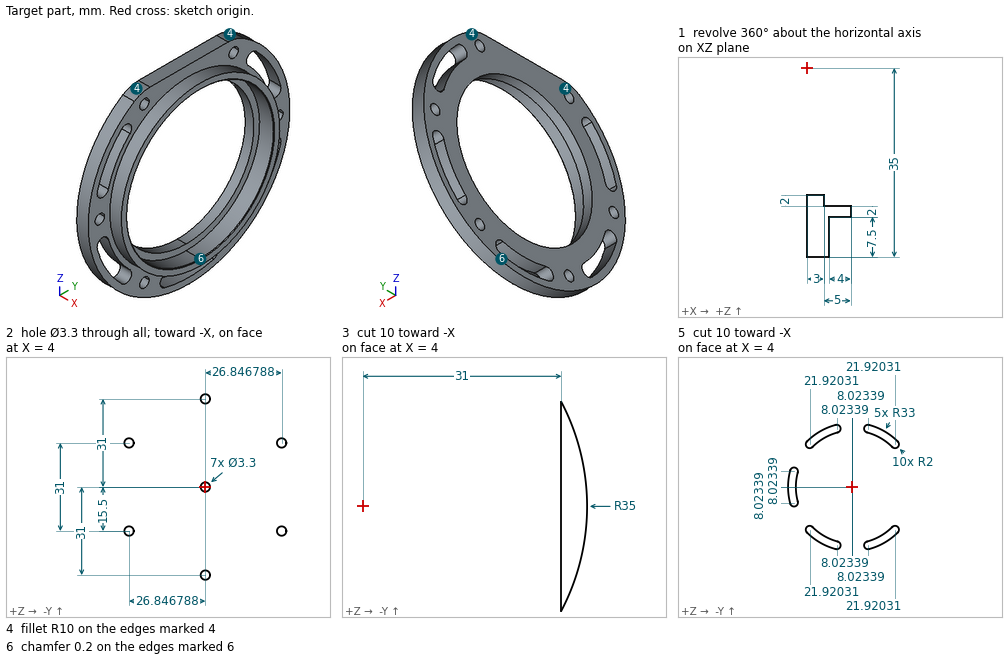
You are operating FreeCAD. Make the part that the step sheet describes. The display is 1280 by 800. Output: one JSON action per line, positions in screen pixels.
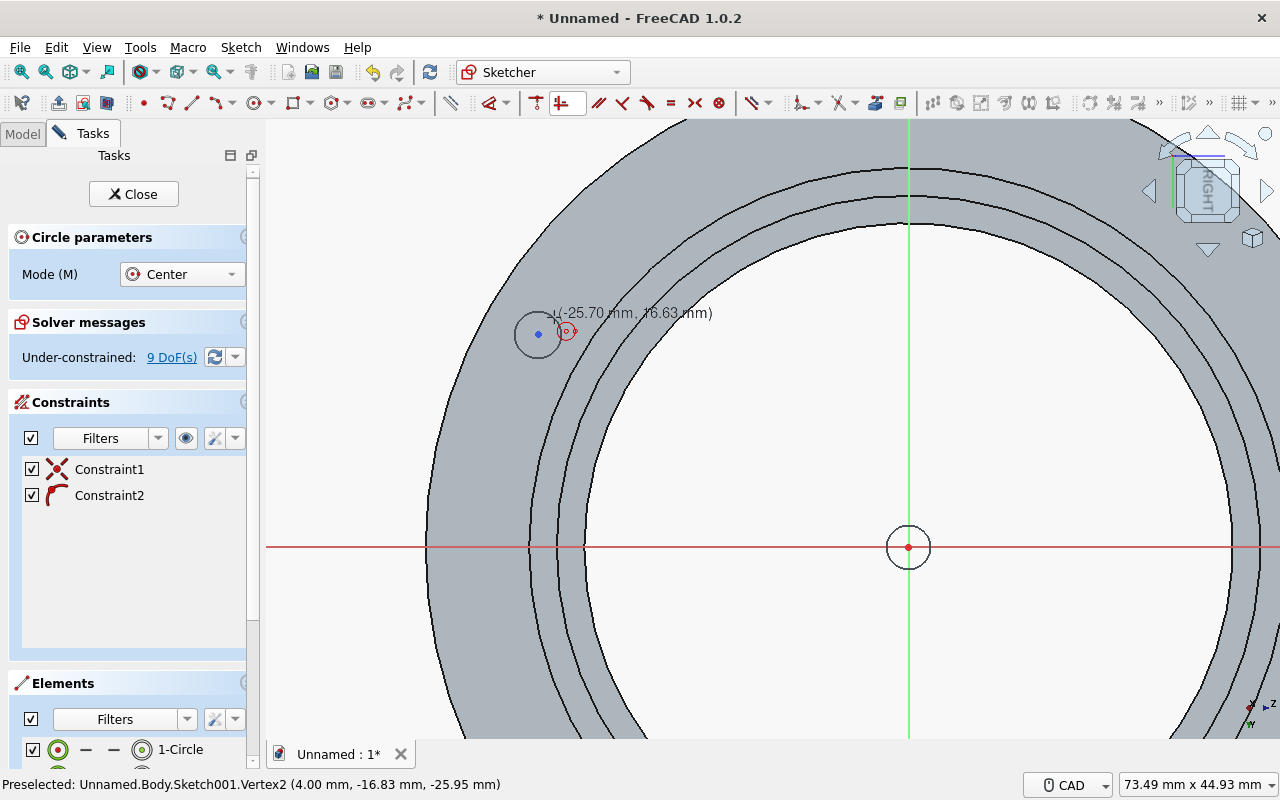
{"action": "scroll", "coordinate": [538, 332], "scroll_direction": "down", "scroll_amount": 4}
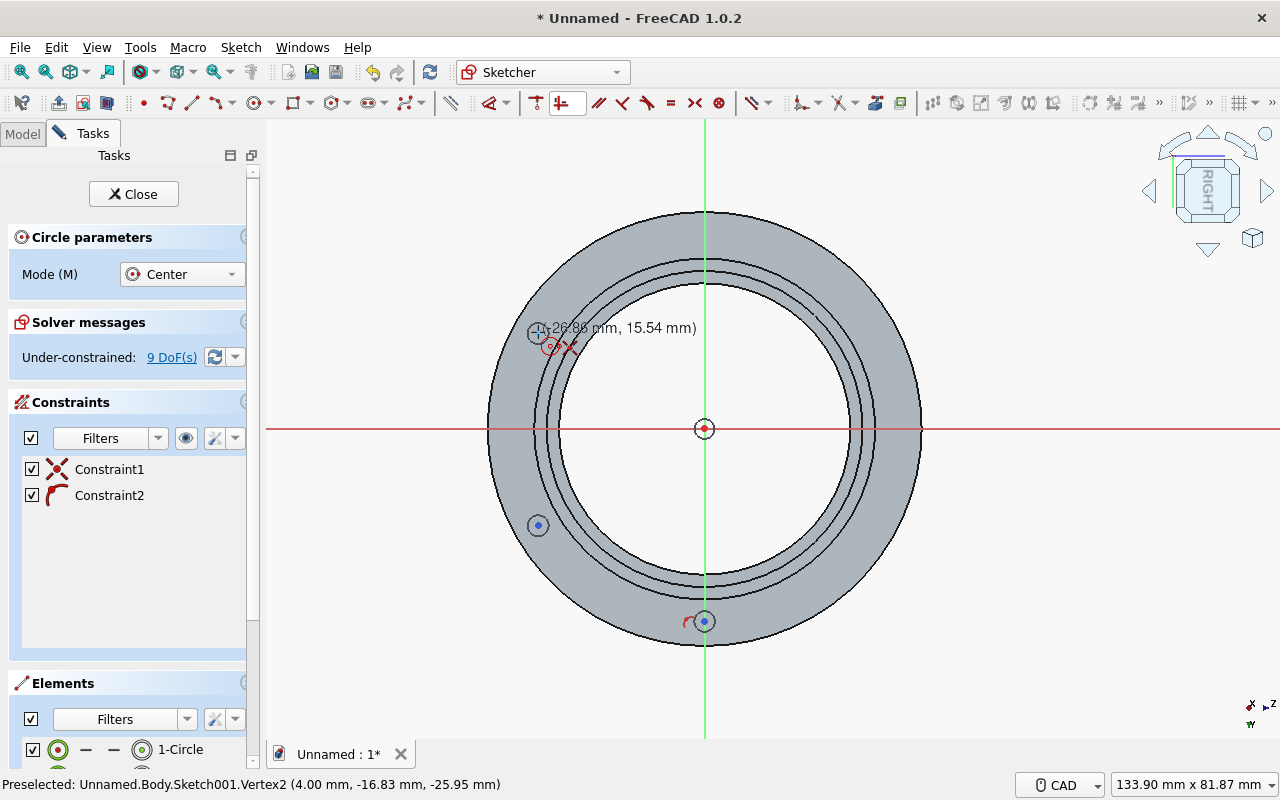
{"action": "scroll", "coordinate": [705, 237], "scroll_direction": "up", "scroll_amount": 4}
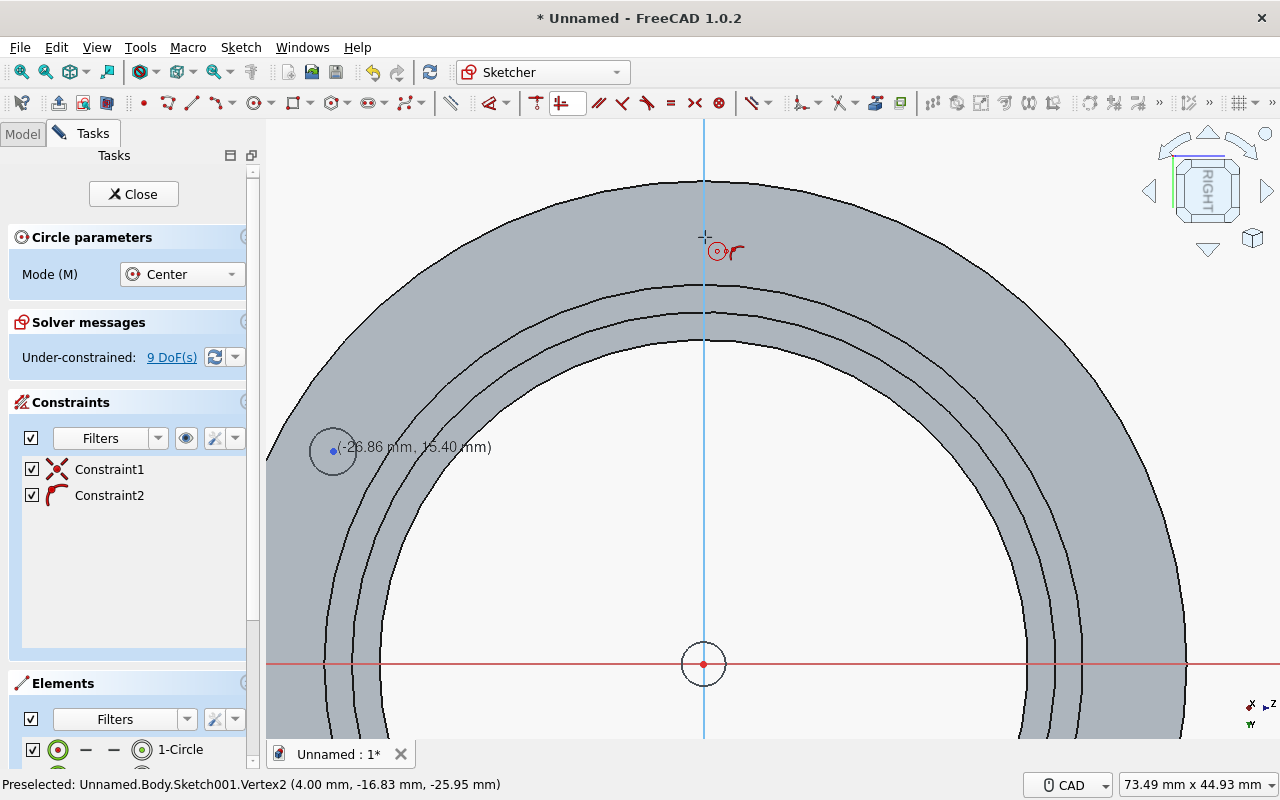
{"action": "left_click", "coordinate": [704, 236]}
{"action": "left_click", "coordinate": [720, 220]}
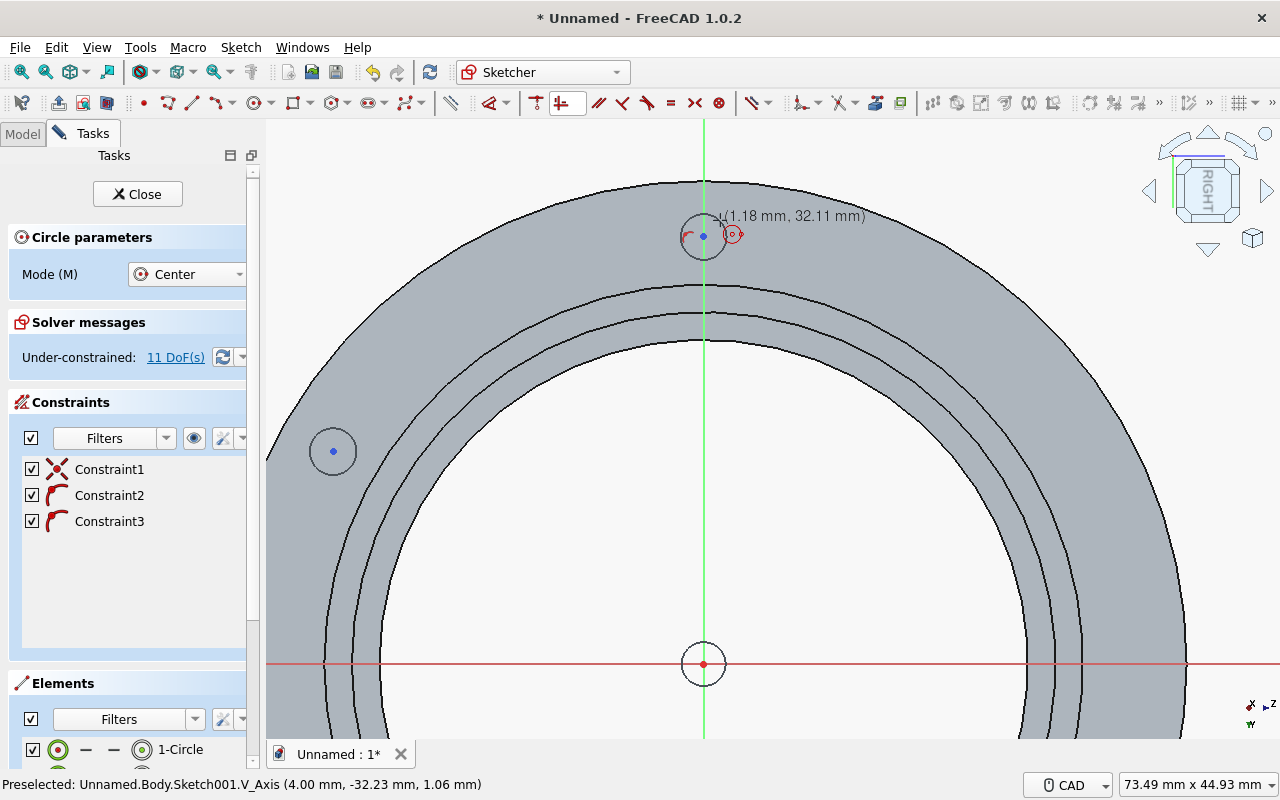
{"action": "left_click", "coordinate": [1074, 450]}
{"action": "left_click", "coordinate": [1090, 434]}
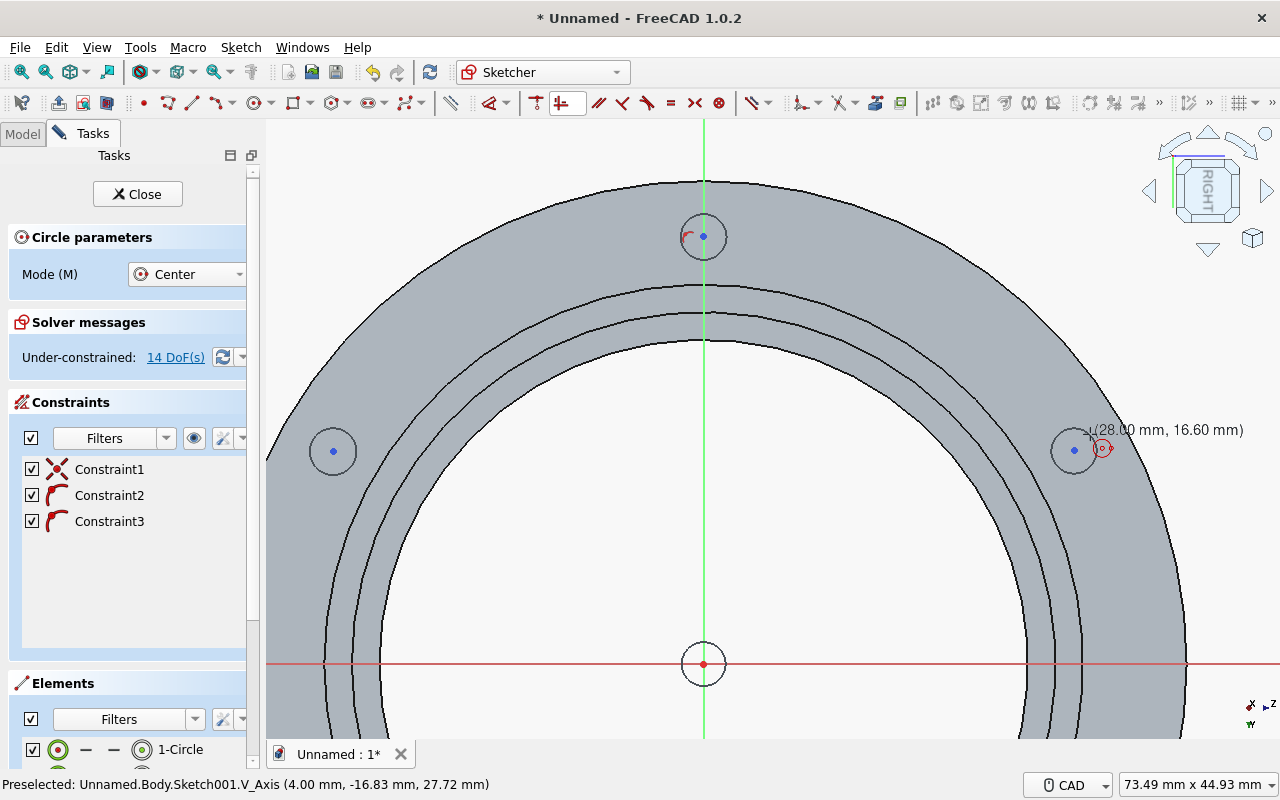
{"action": "scroll", "coordinate": [705, 237], "scroll_direction": "down", "scroll_amount": 4}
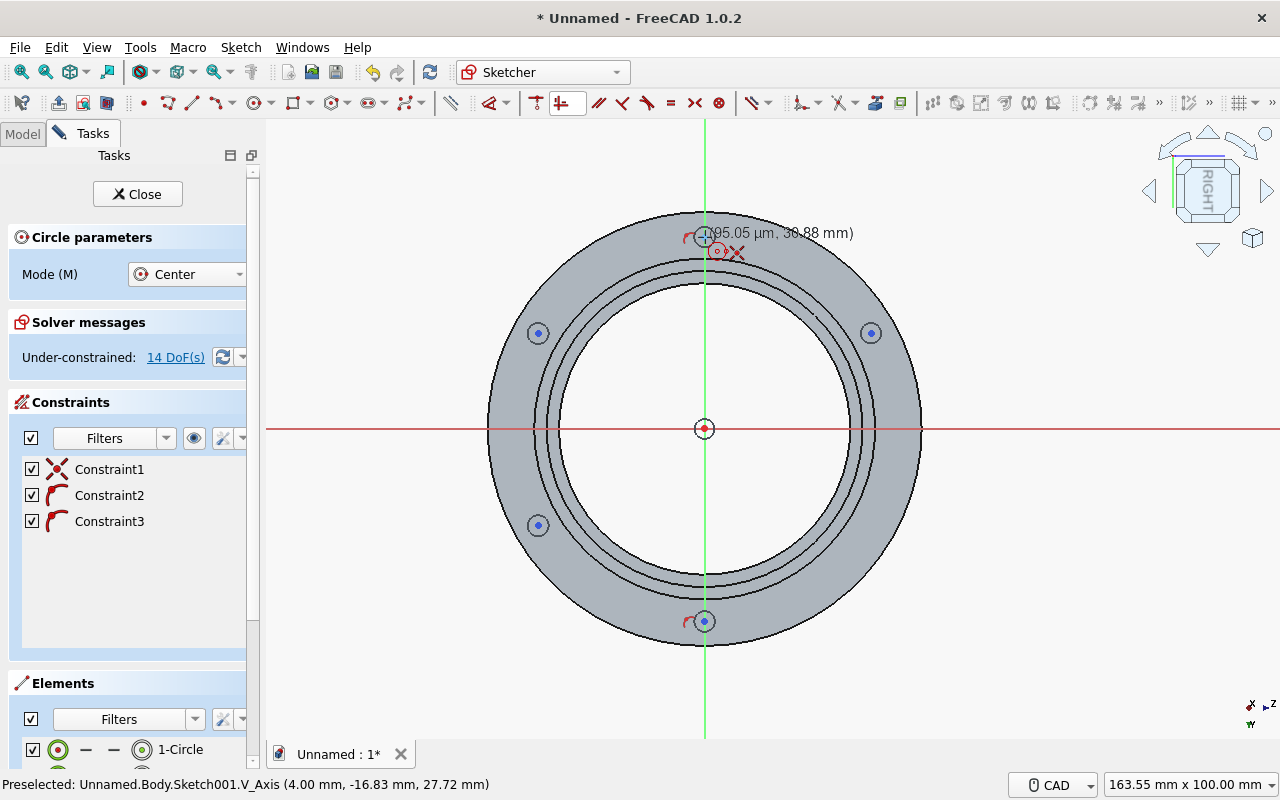
{"action": "scroll", "coordinate": [871, 525], "scroll_direction": "up", "scroll_amount": 4}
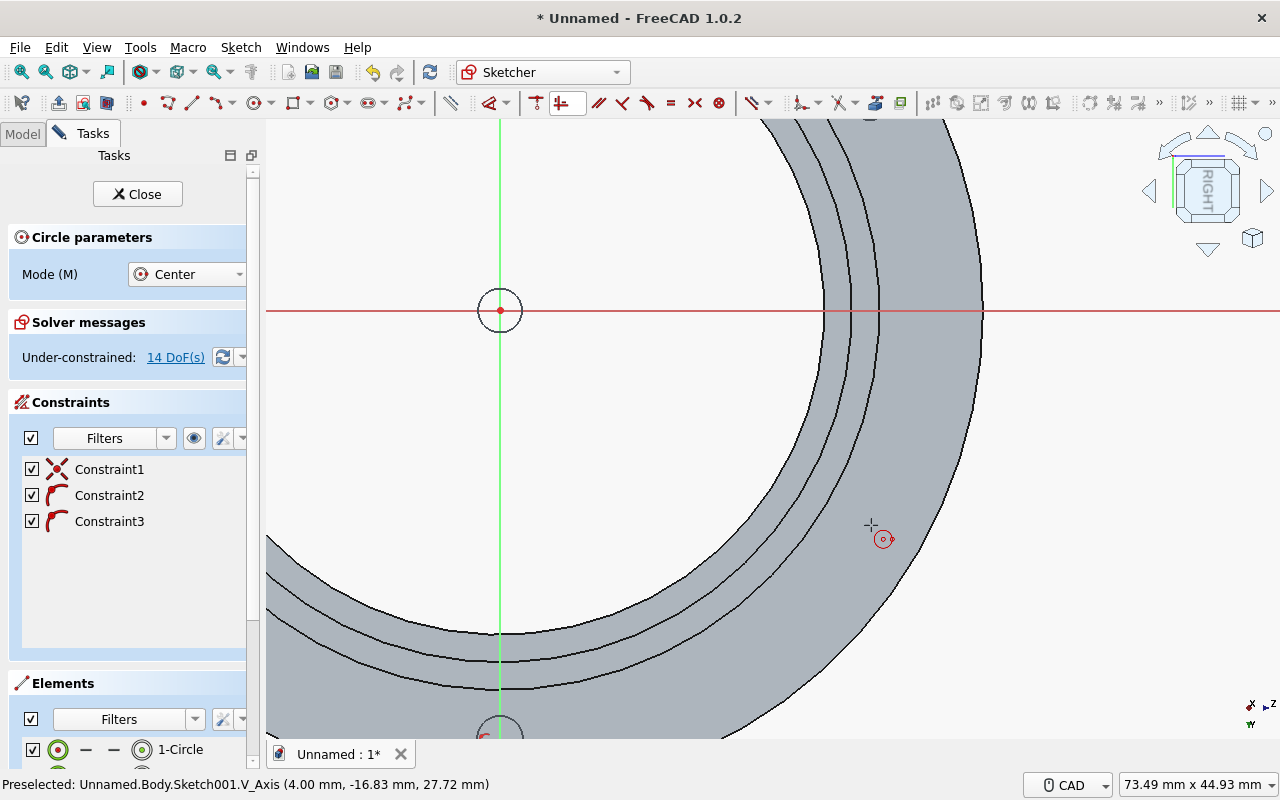
{"action": "left_click", "coordinate": [870, 524]}
{"action": "left_click", "coordinate": [887, 508]}
{"action": "key", "text": "Escape"}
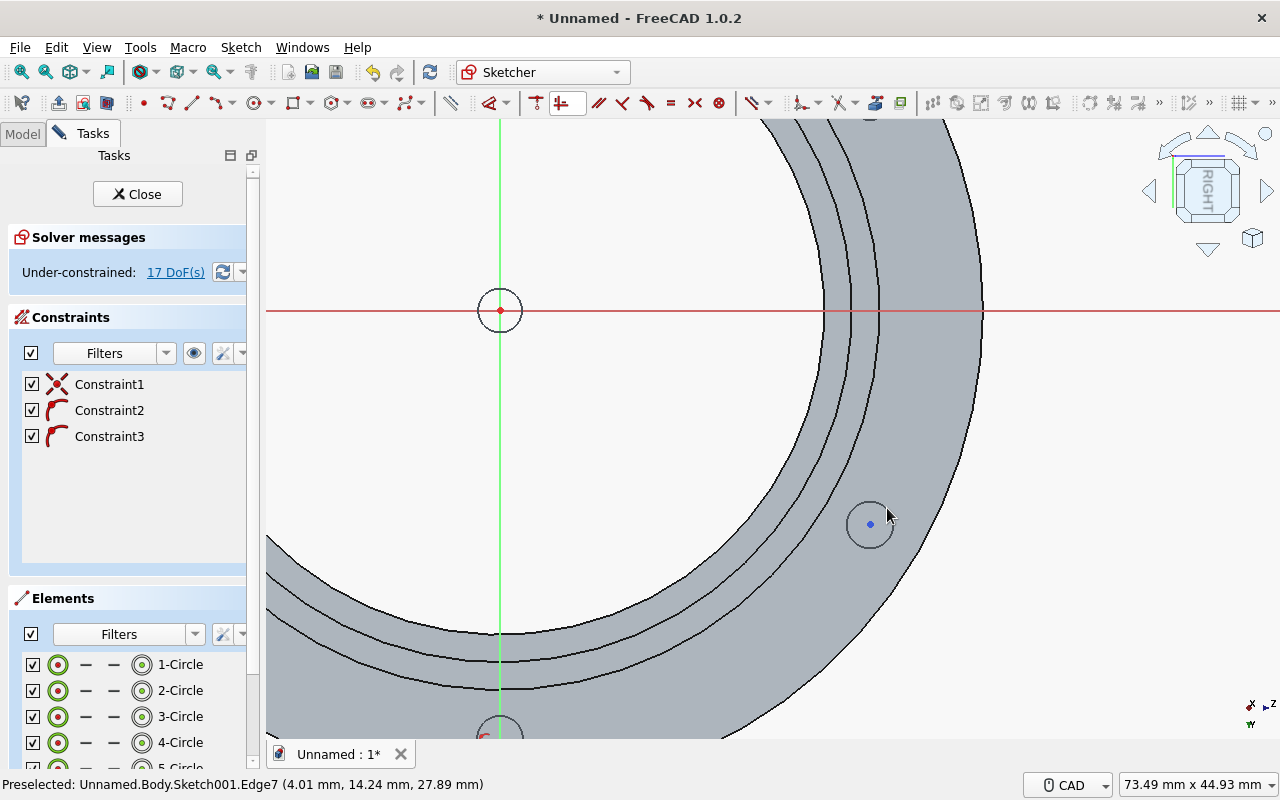
{"action": "left_click", "coordinate": [515, 295]}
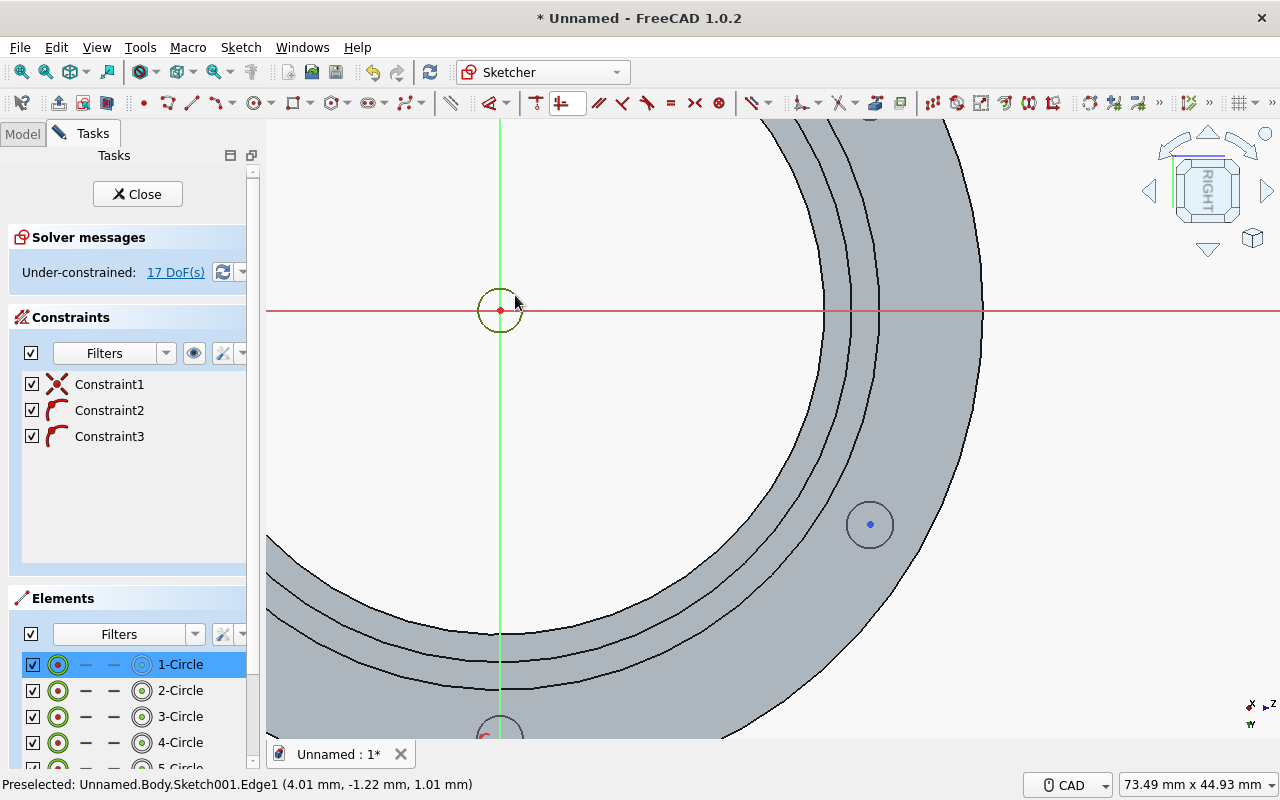
{"action": "scroll", "coordinate": [871, 526], "scroll_direction": "down", "scroll_amount": 4}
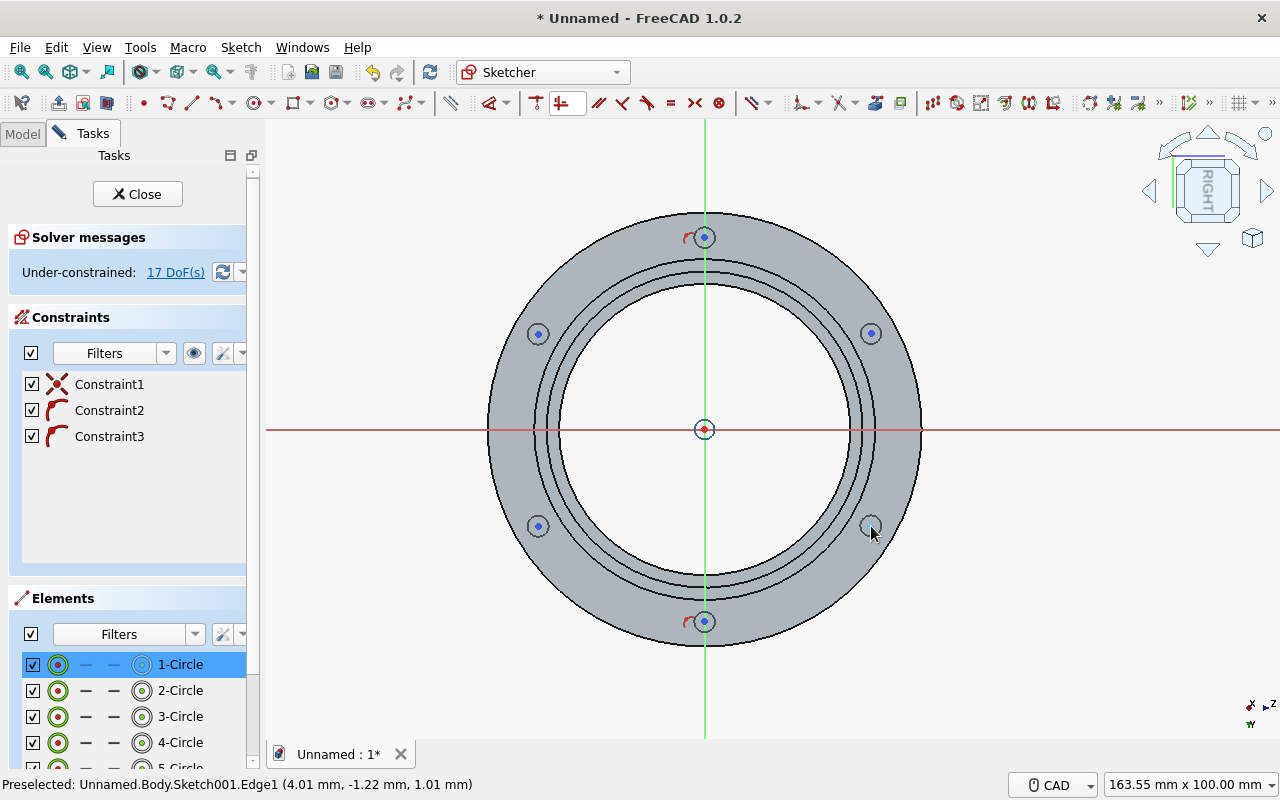
{"action": "scroll", "coordinate": [712, 615], "scroll_direction": "up", "scroll_amount": 4}